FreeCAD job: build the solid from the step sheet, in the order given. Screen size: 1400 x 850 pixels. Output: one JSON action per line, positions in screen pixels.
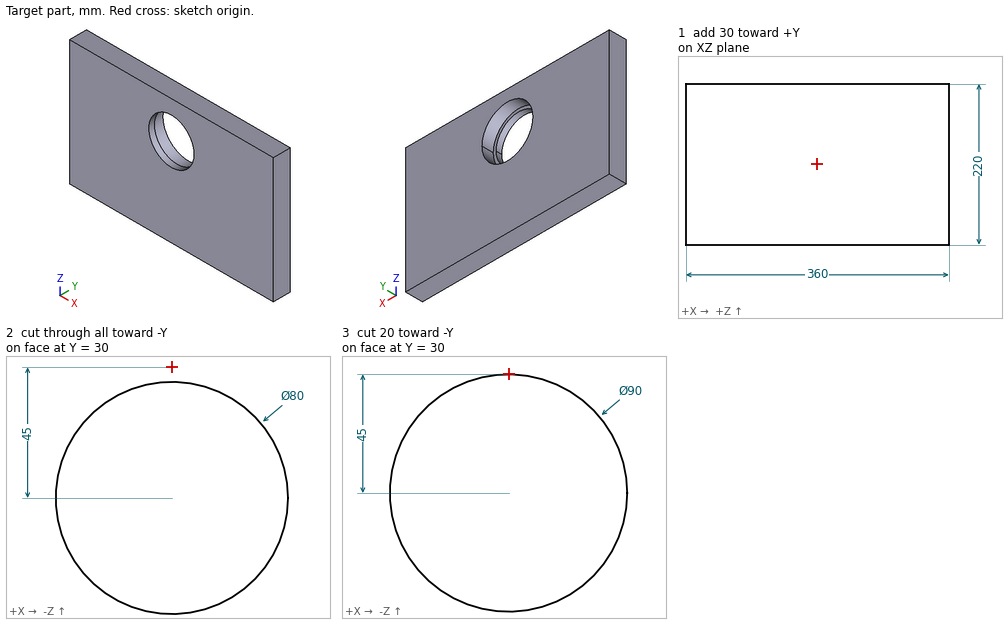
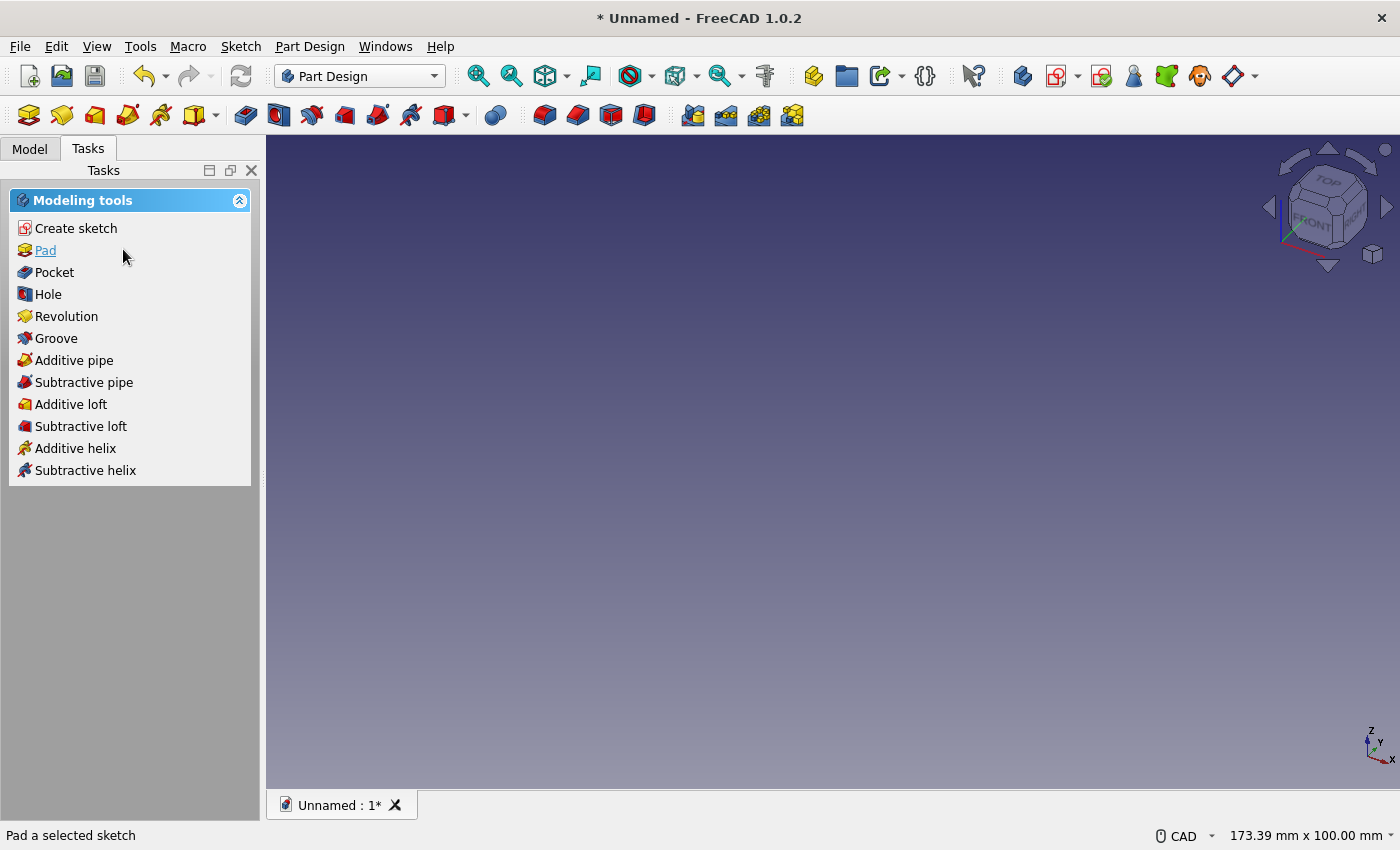
{"action": "left_click", "coordinate": [29, 116]}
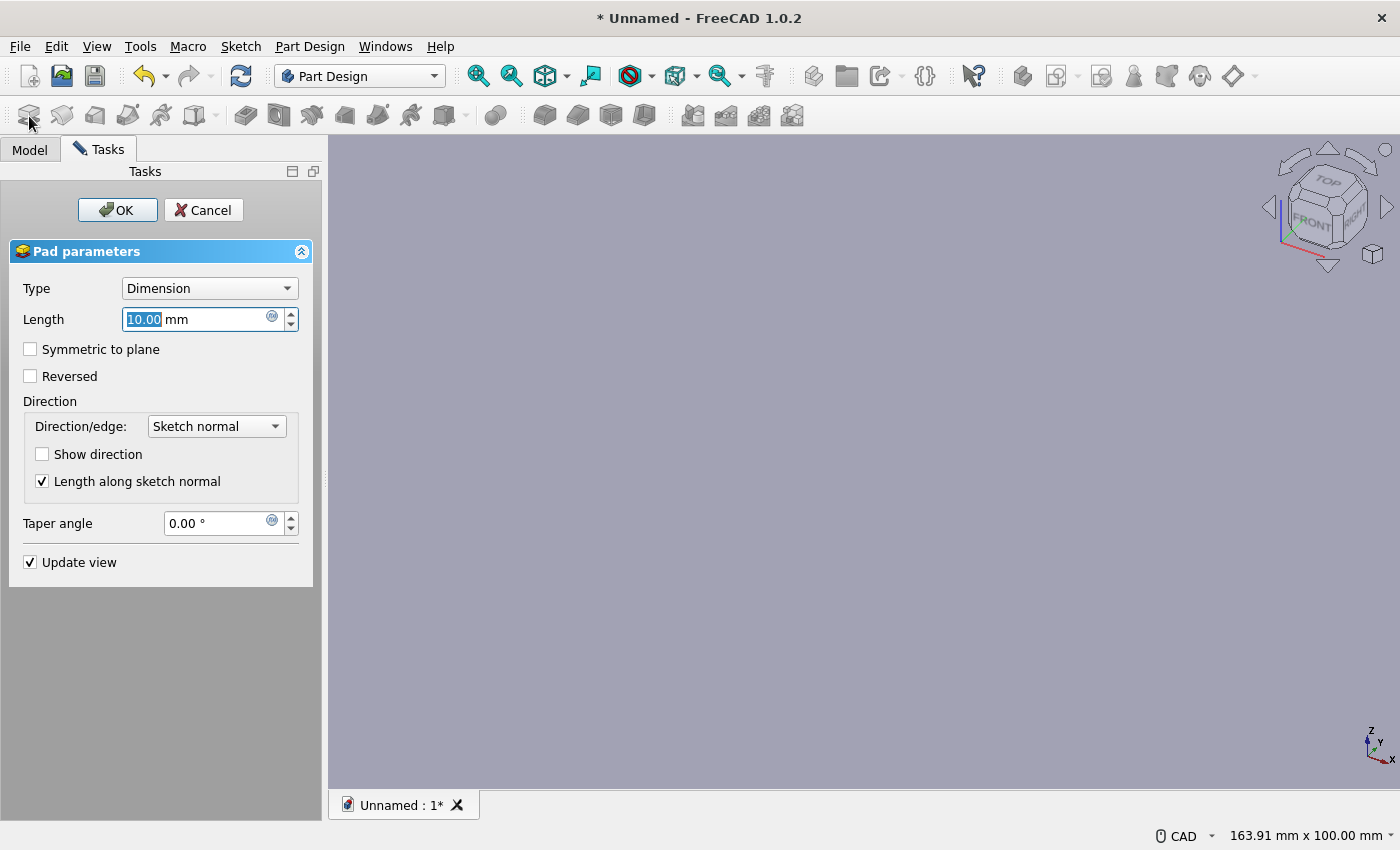
{"action": "type", "text": "30"}
{"action": "key", "text": "Tab"}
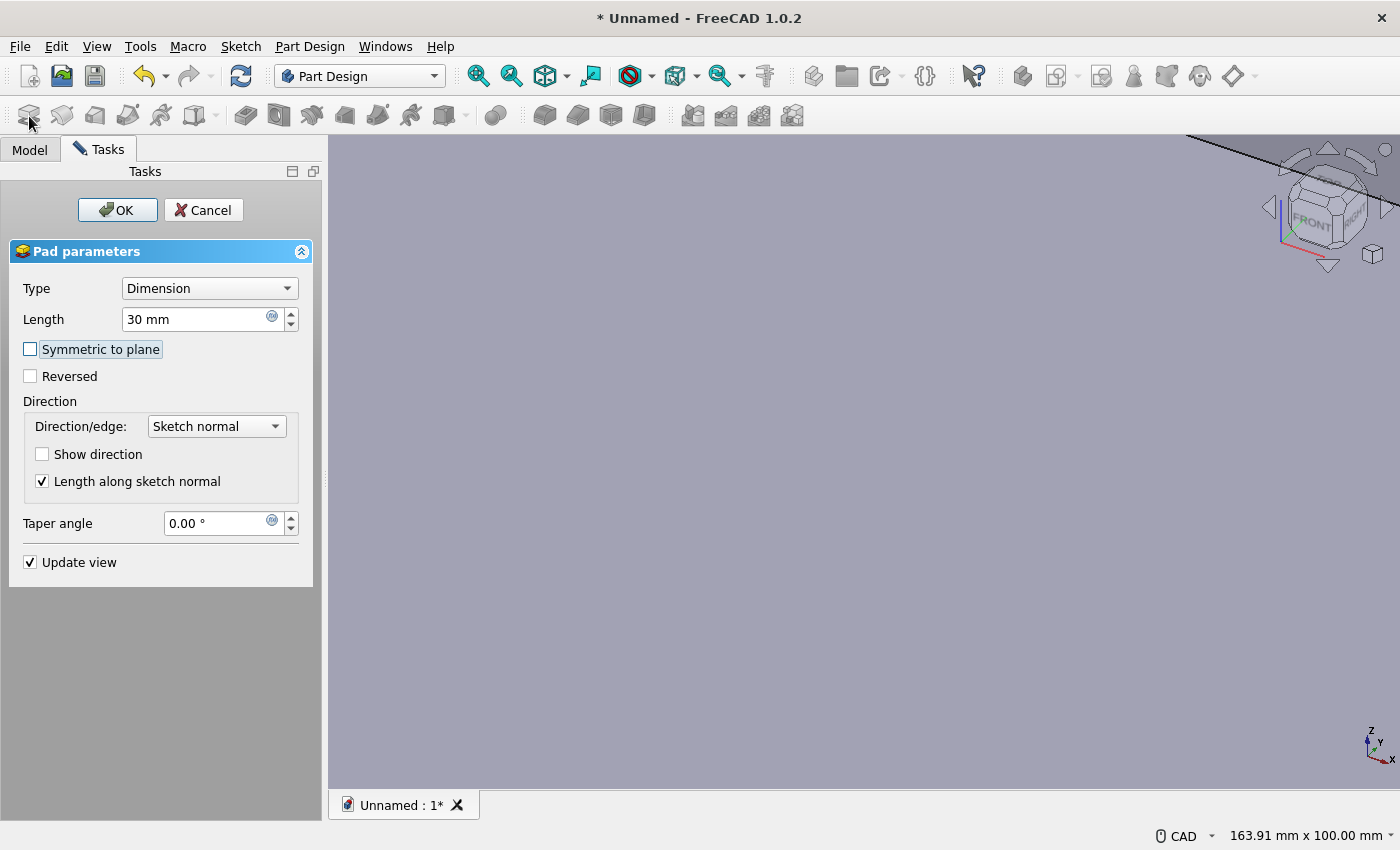
{"action": "left_click", "coordinate": [31, 376]}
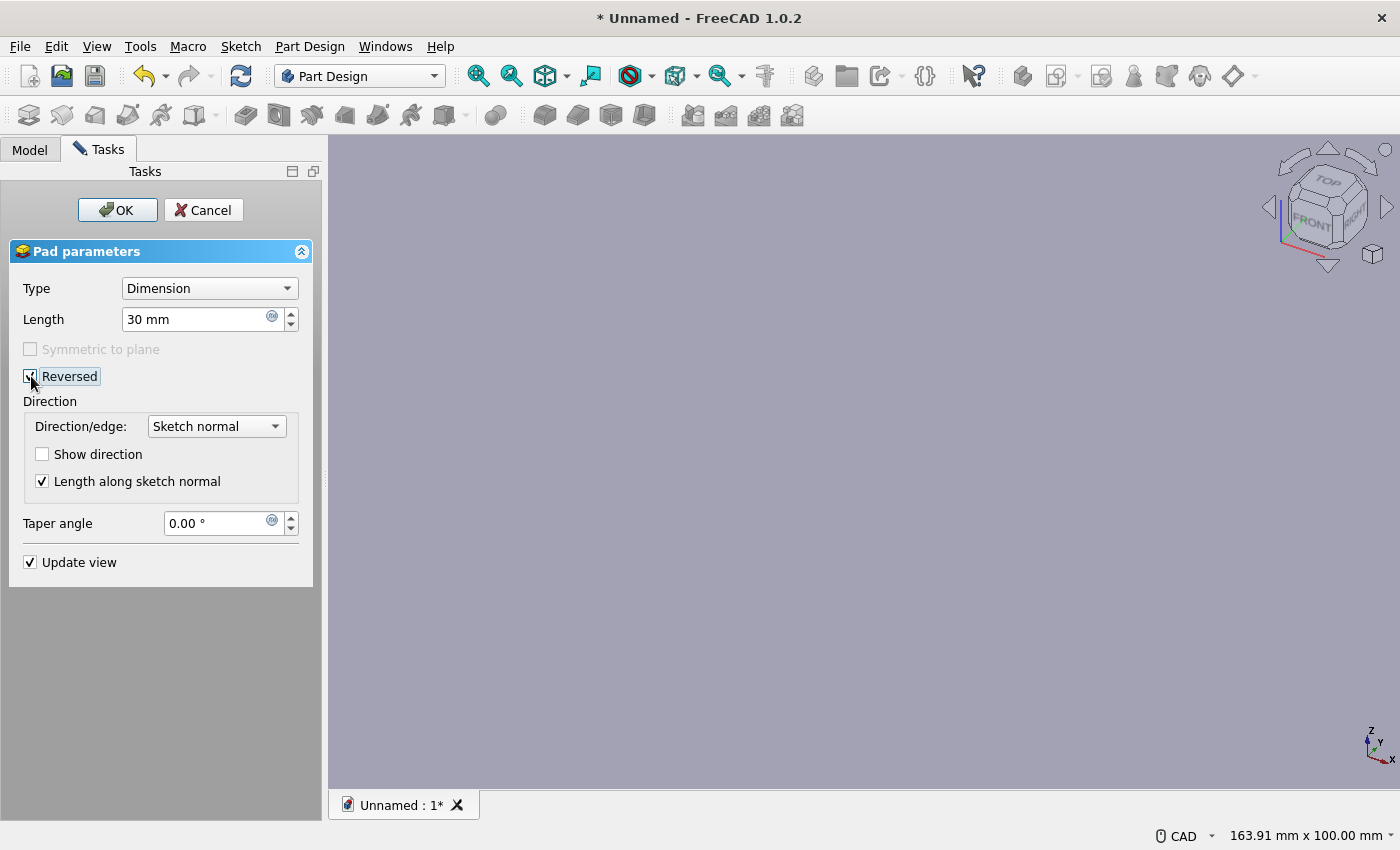
{"action": "left_click", "coordinate": [118, 210]}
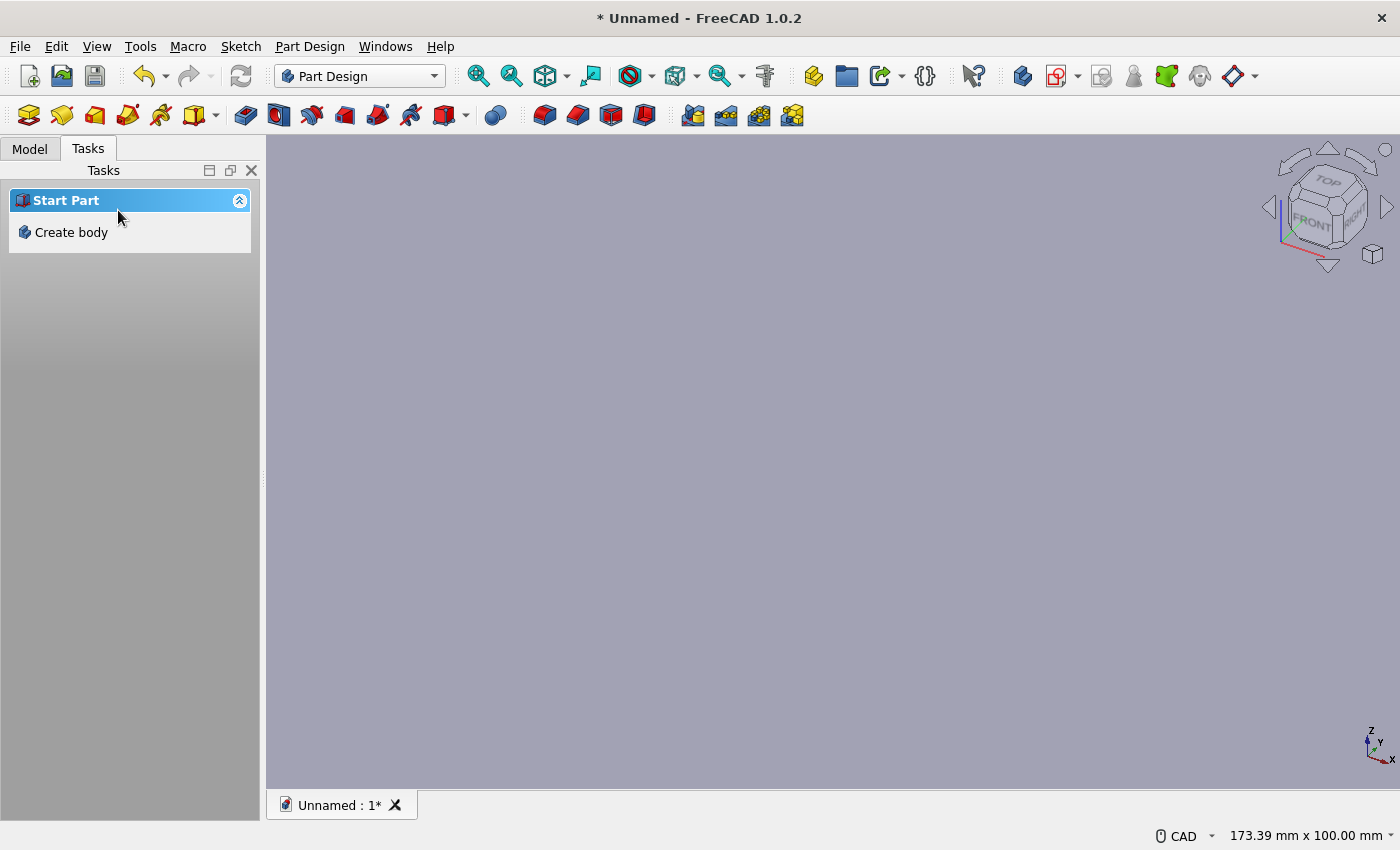
{"action": "left_click", "coordinate": [479, 76]}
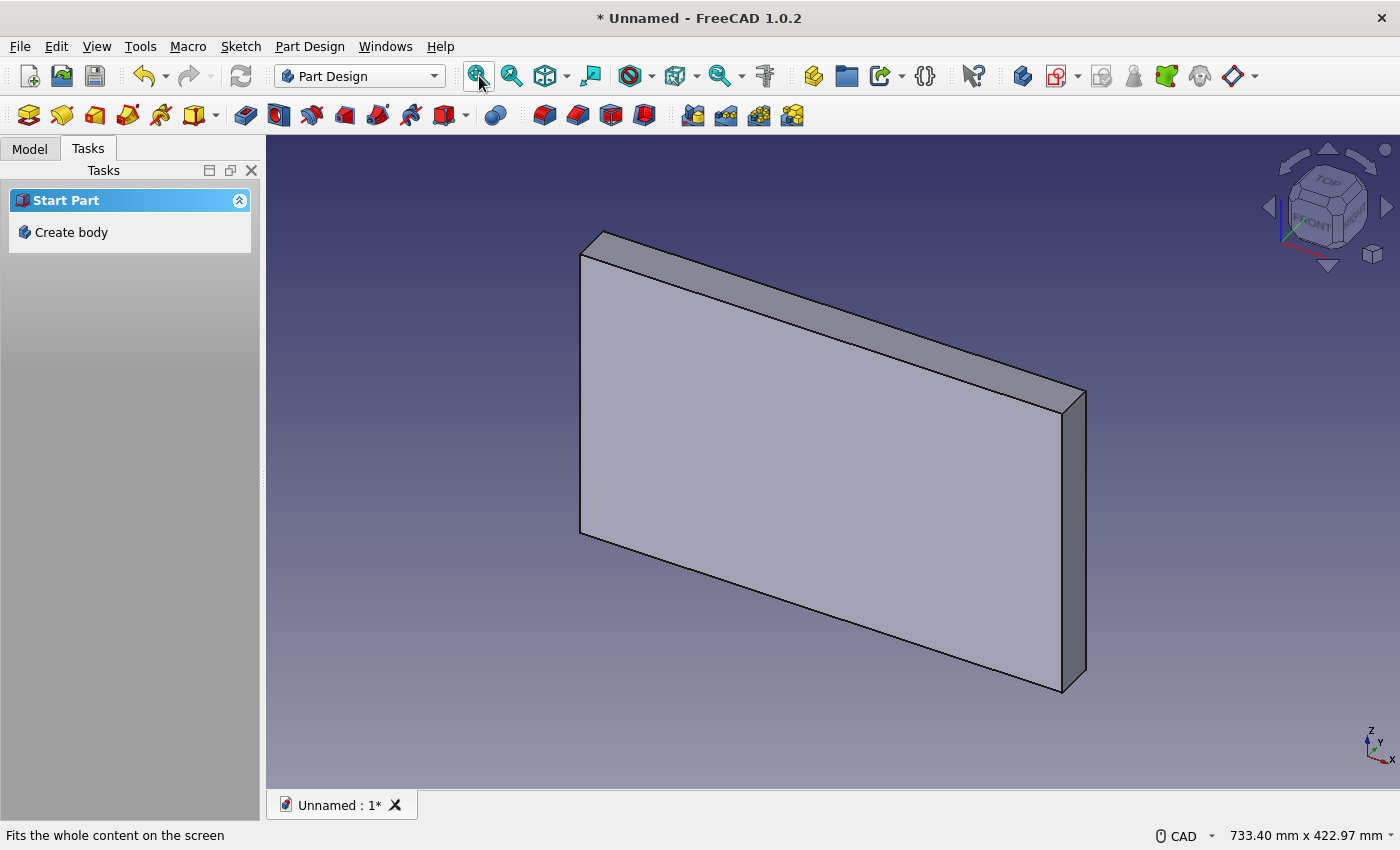
{"action": "key", "text": "4"}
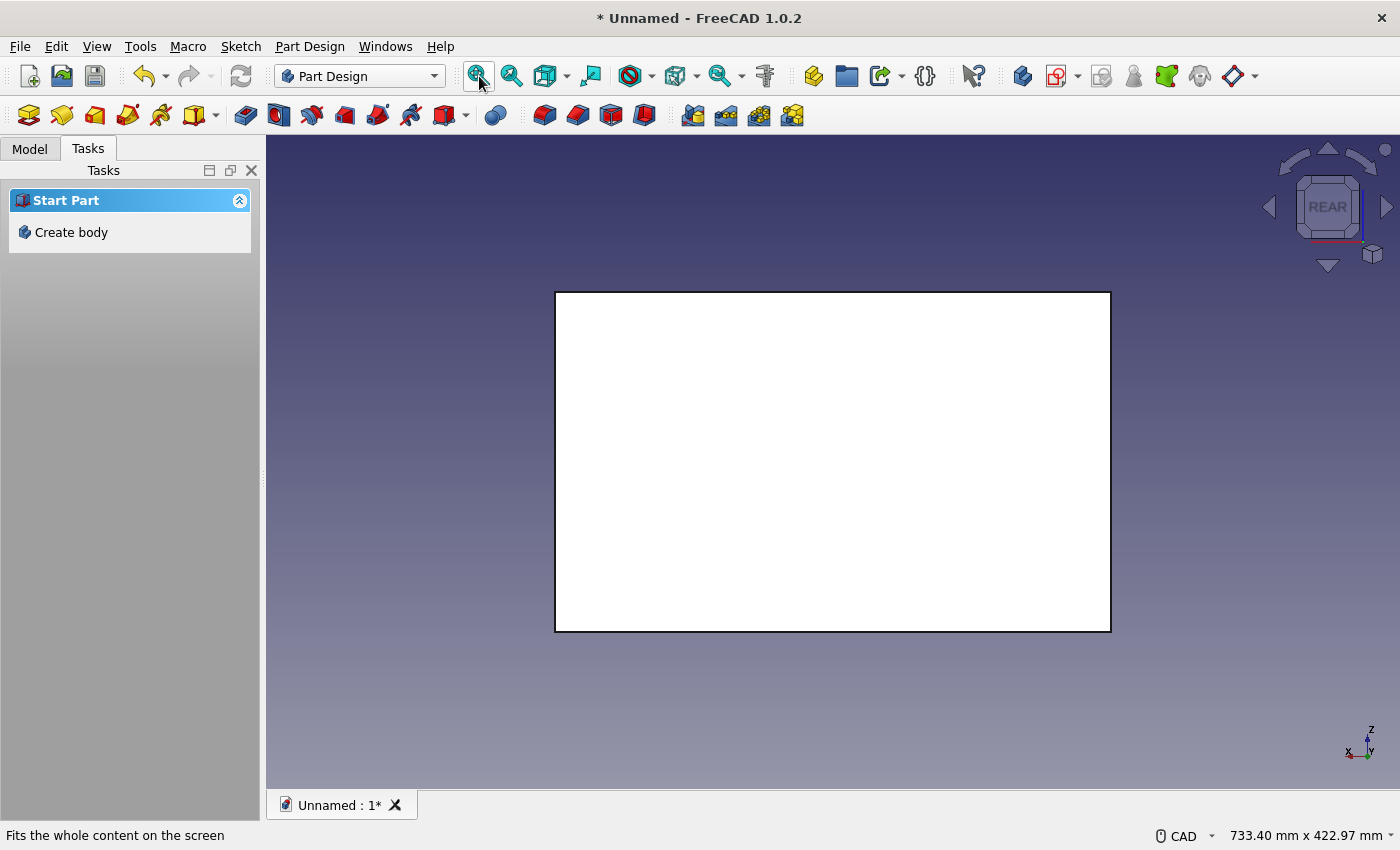
{"action": "left_click", "coordinate": [753, 461]}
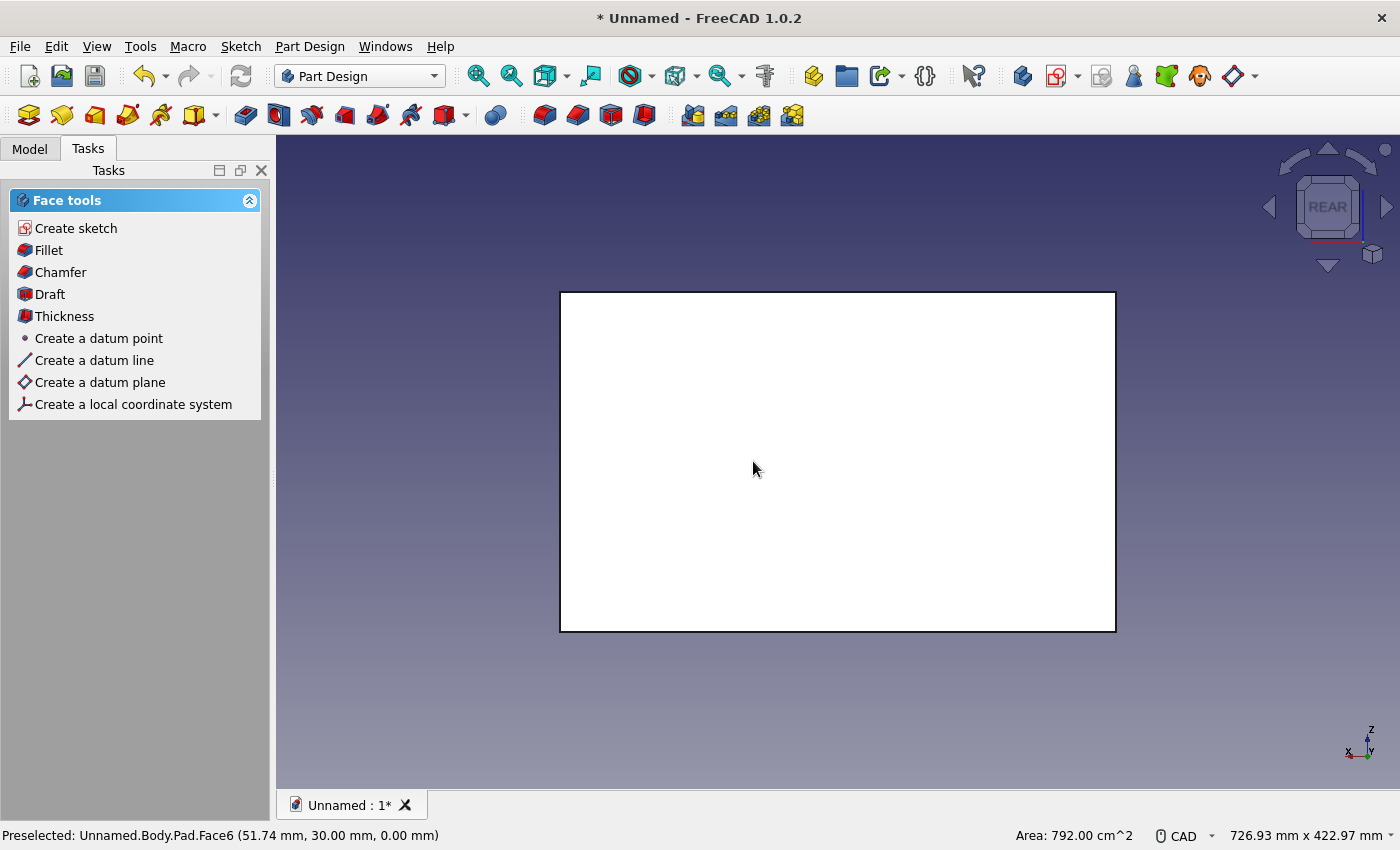
{"action": "left_click", "coordinate": [1056, 76]}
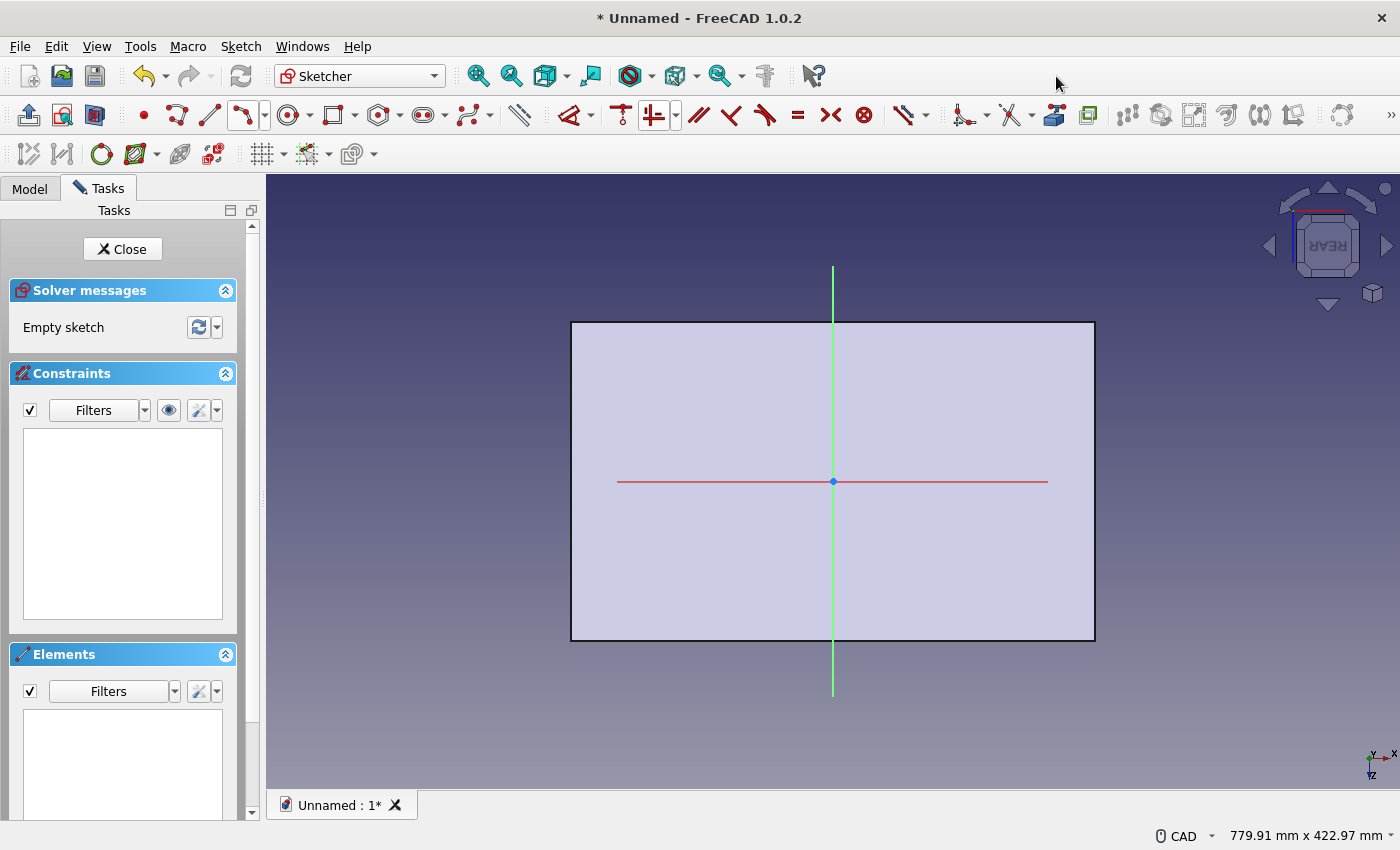
{"action": "scroll", "coordinate": [863, 570], "scroll_direction": "up", "scroll_amount": 6}